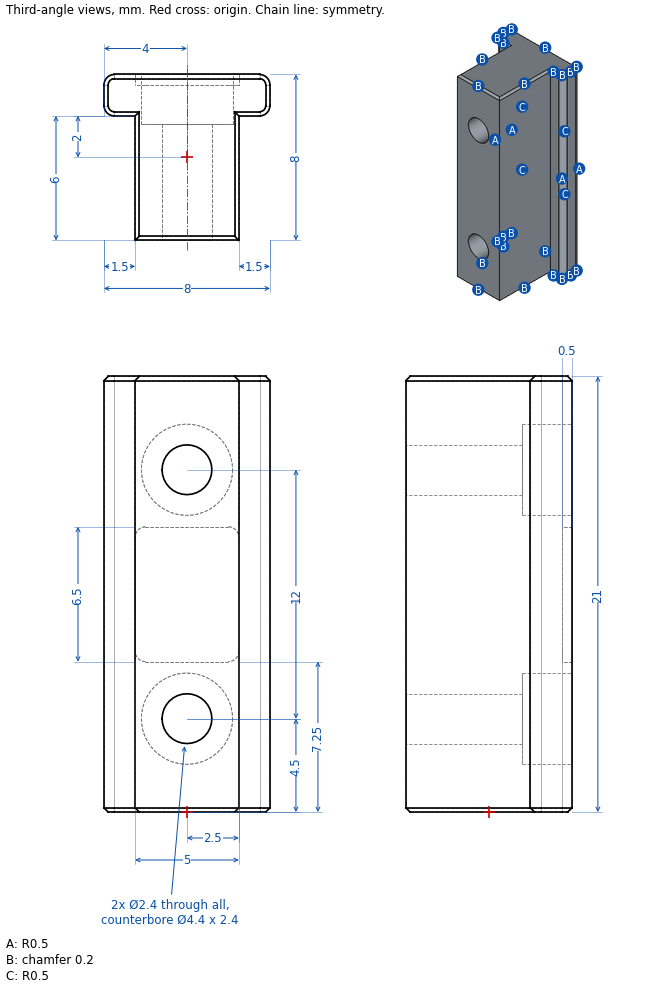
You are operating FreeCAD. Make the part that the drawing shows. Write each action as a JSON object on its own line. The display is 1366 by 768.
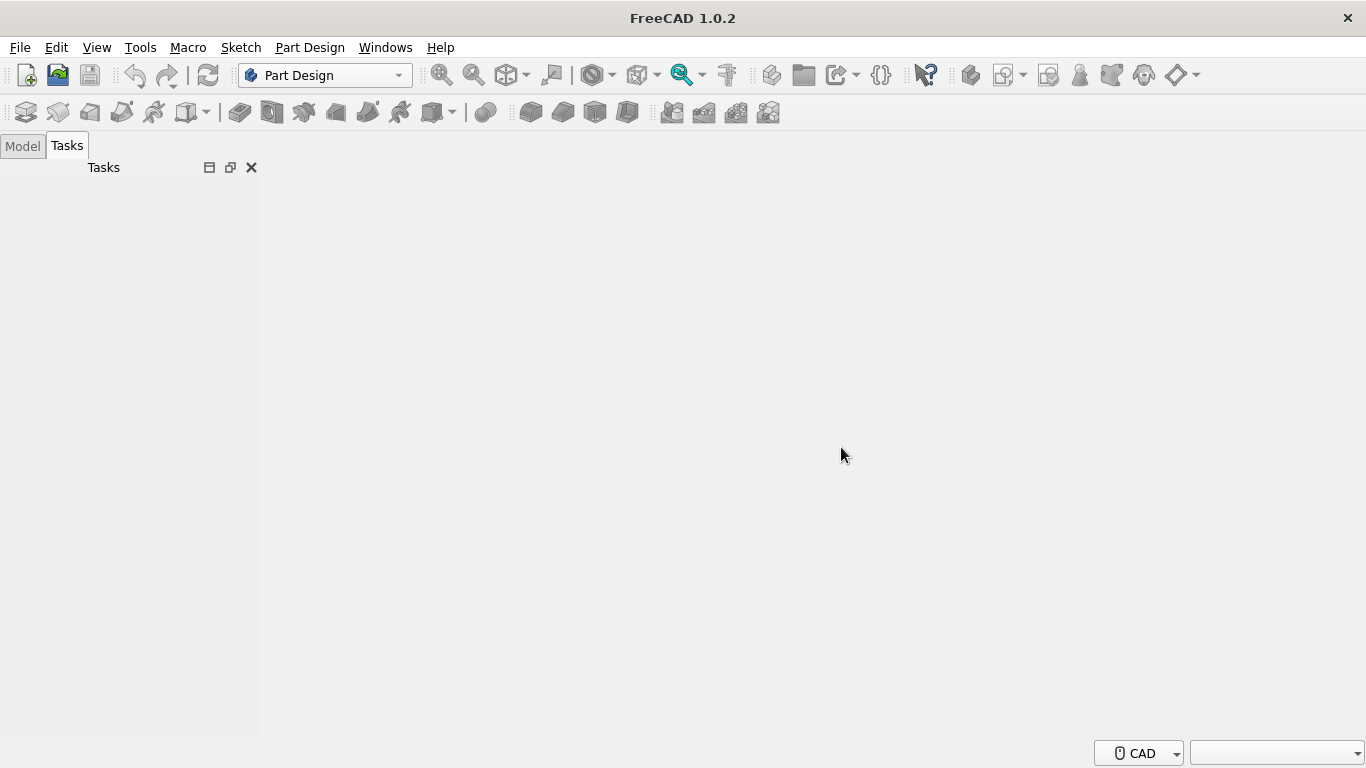
{"action": "left_click", "coordinate": [26, 76]}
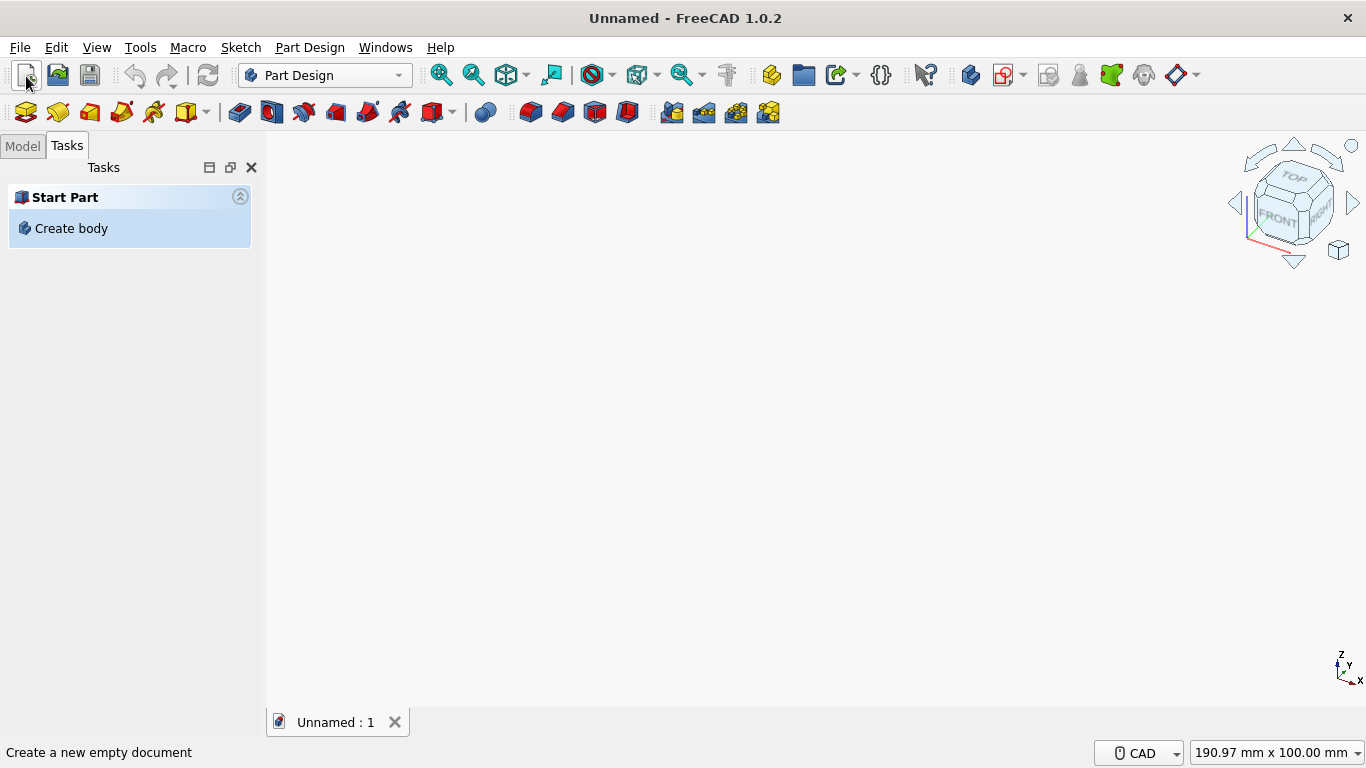
{"action": "left_click", "coordinate": [1004, 76]}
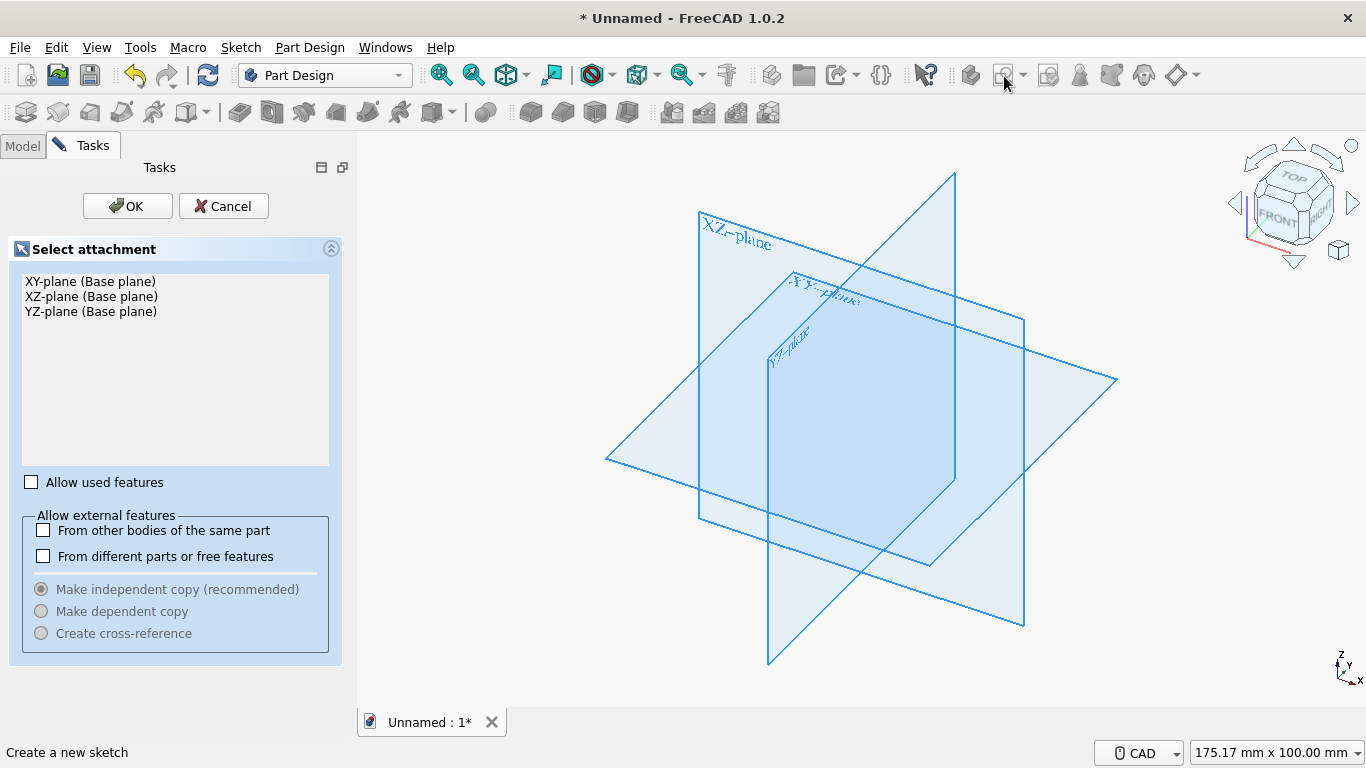
{"action": "left_click", "coordinate": [82, 282]}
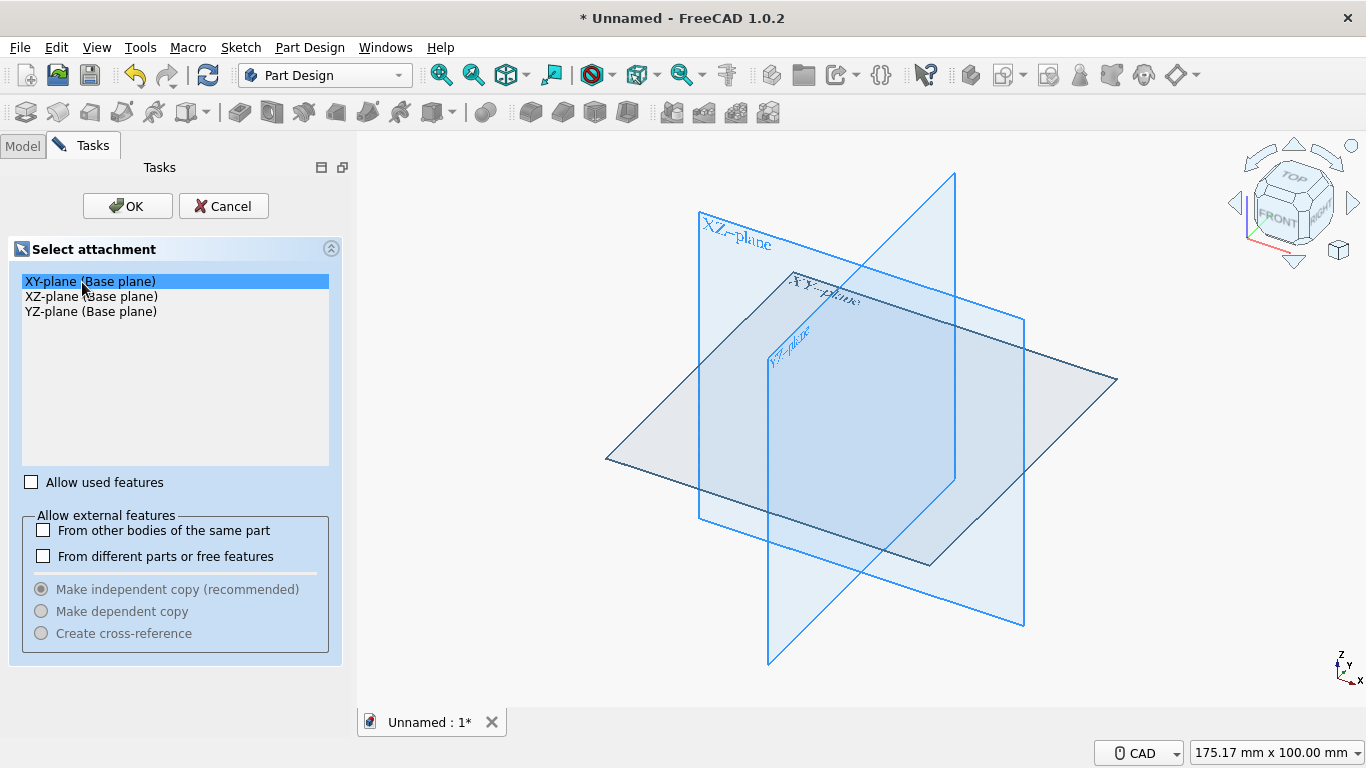
{"action": "left_click", "coordinate": [128, 206]}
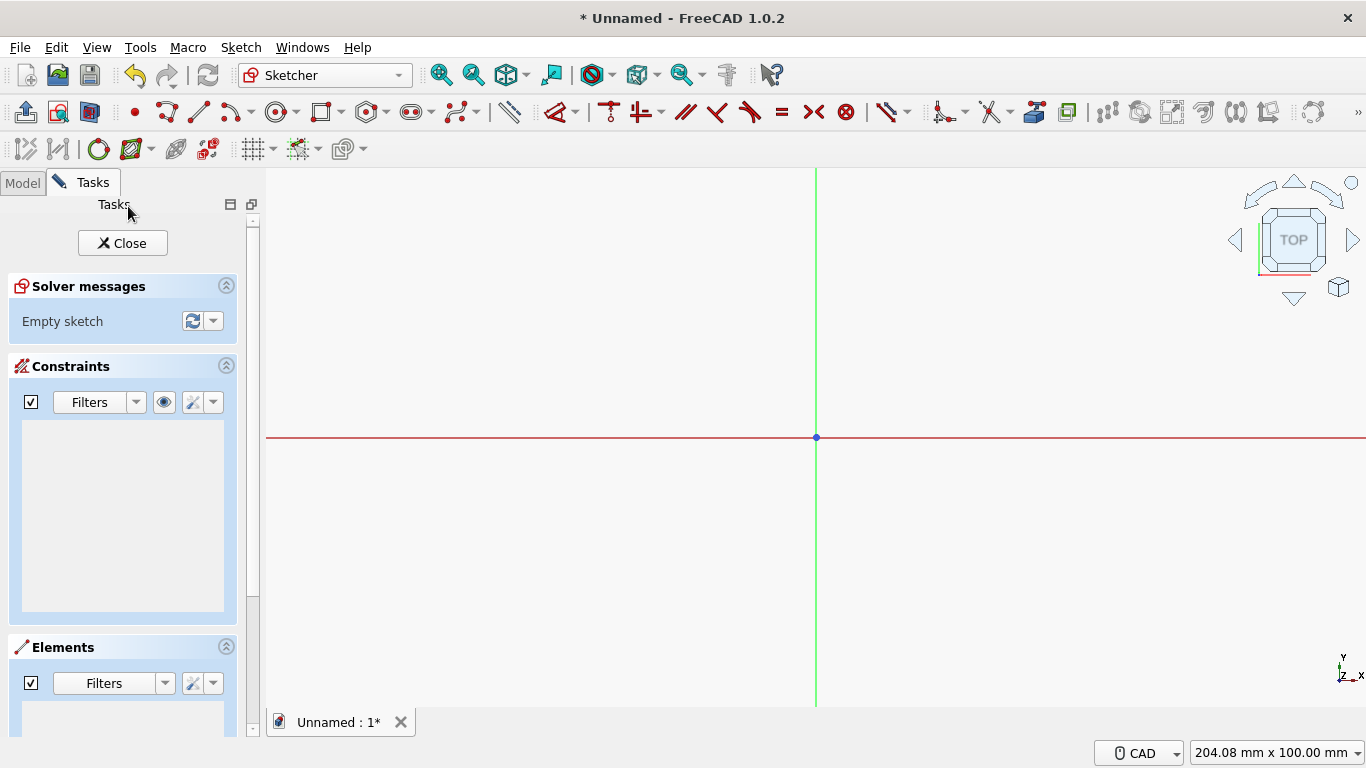
{"action": "scroll", "coordinate": [827, 437], "scroll_direction": "up", "scroll_amount": 10}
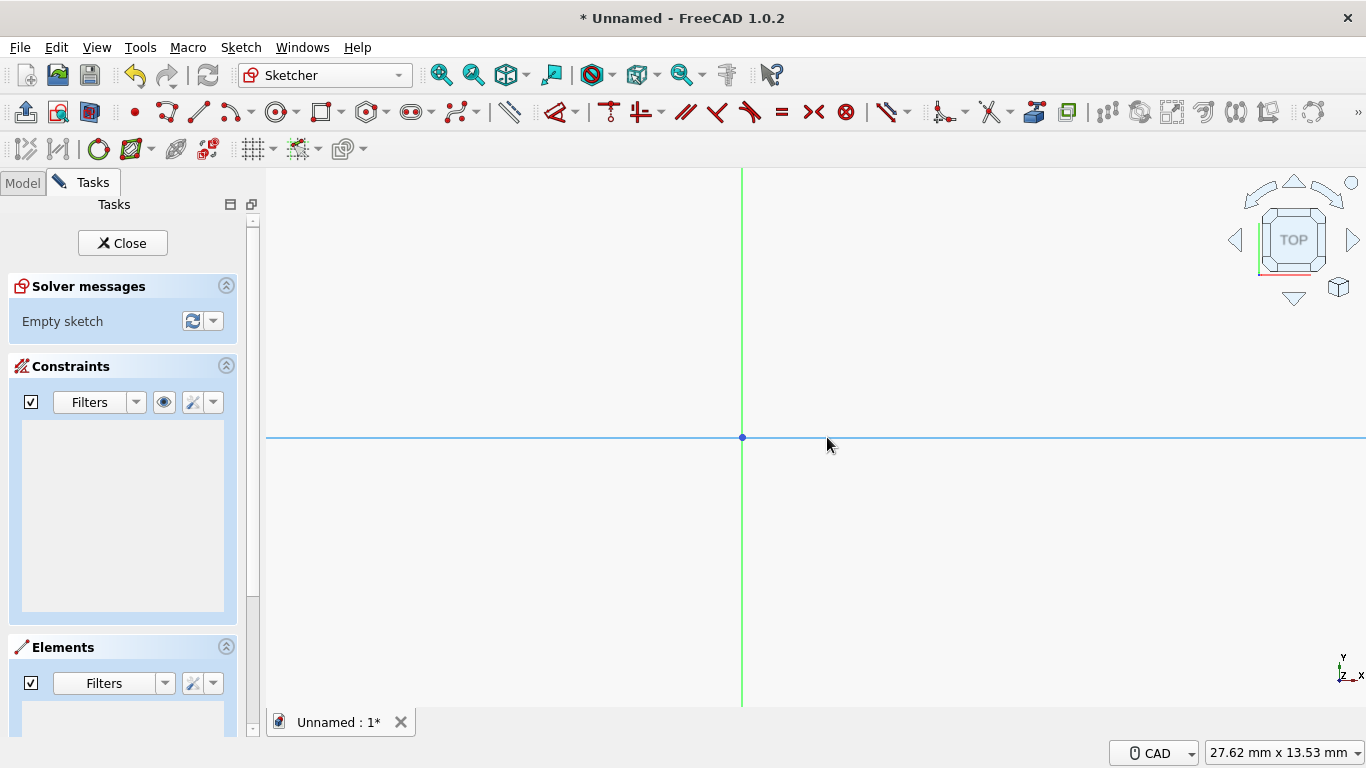
{"action": "key", "text": "g v"}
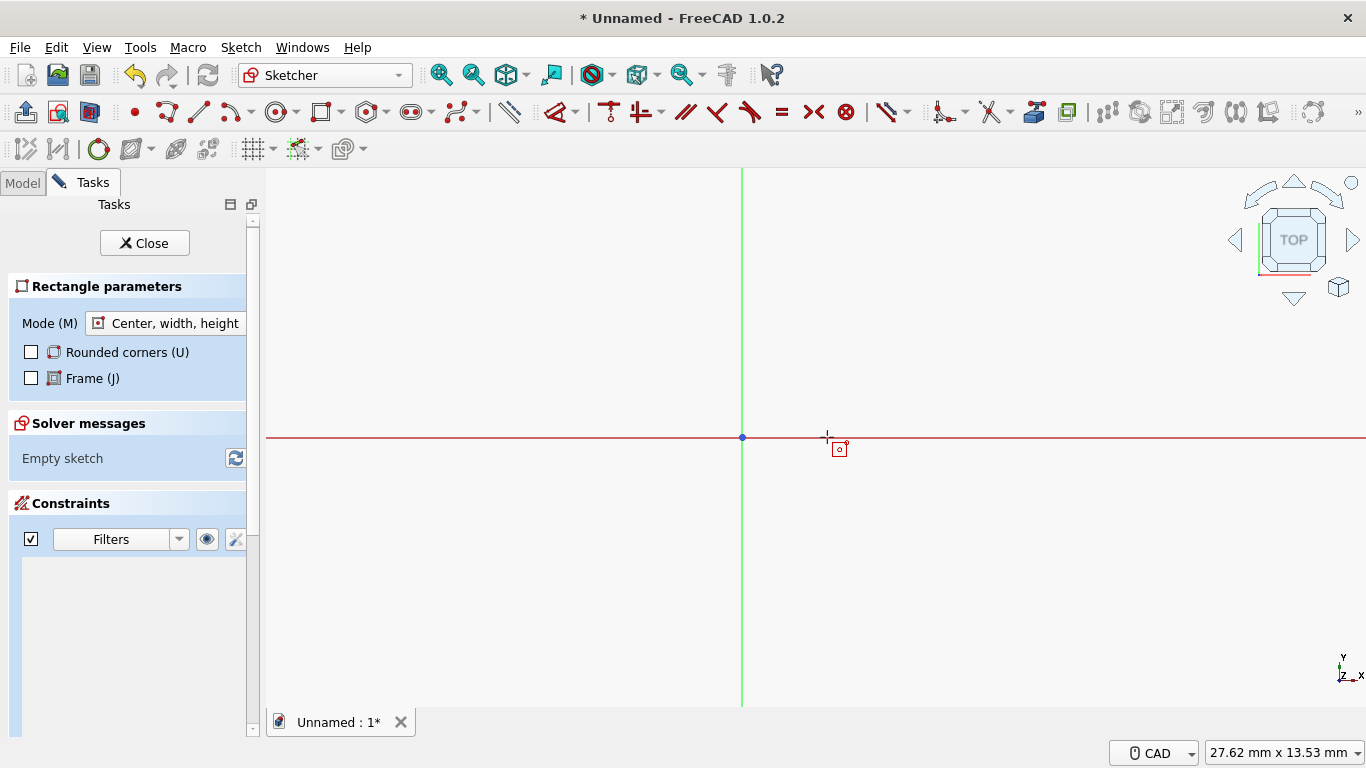
{"action": "left_click", "coordinate": [742, 438]}
{"action": "mouse_move", "coordinate": [902, 278]}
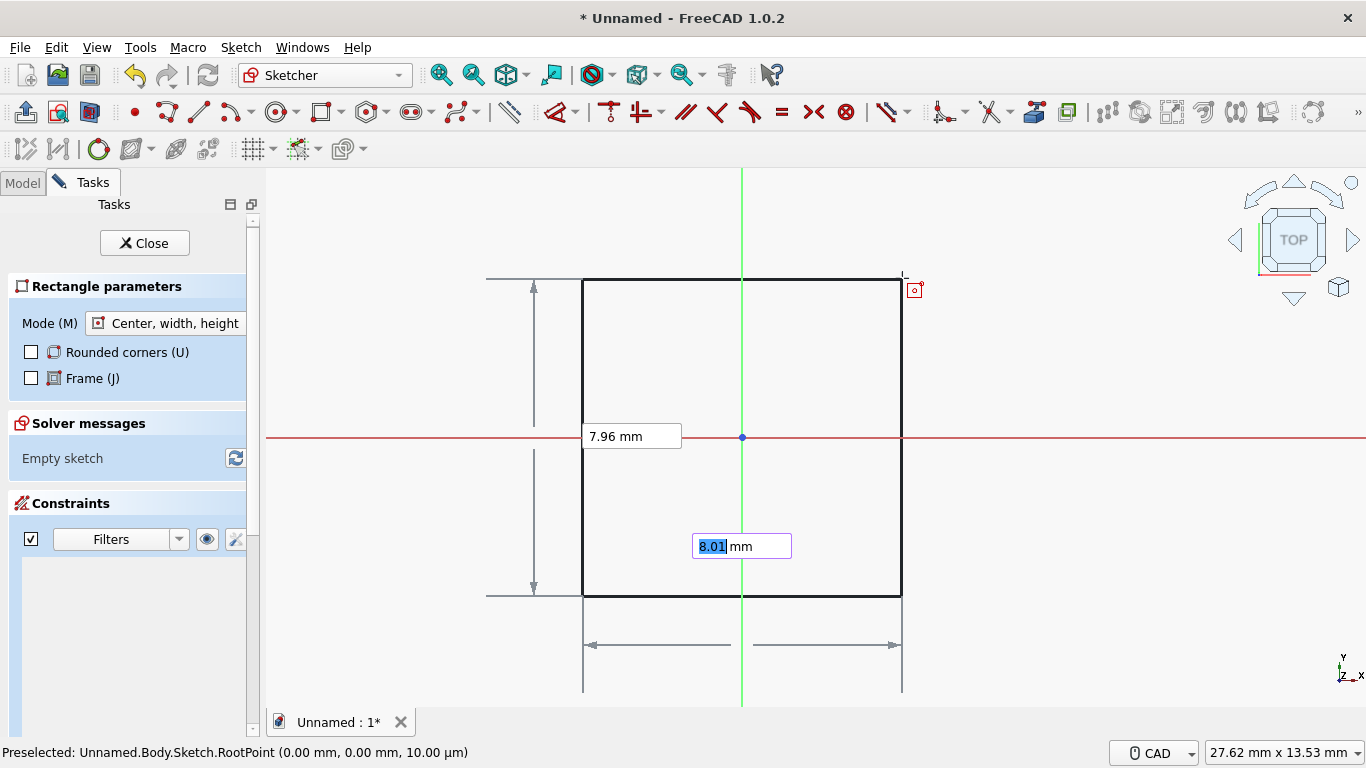
{"action": "type", "text": "8"}
{"action": "key", "text": "Tab"}
{"action": "type", "text": "8"}
{"action": "key", "text": "Return"}
{"action": "key", "text": "Escape"}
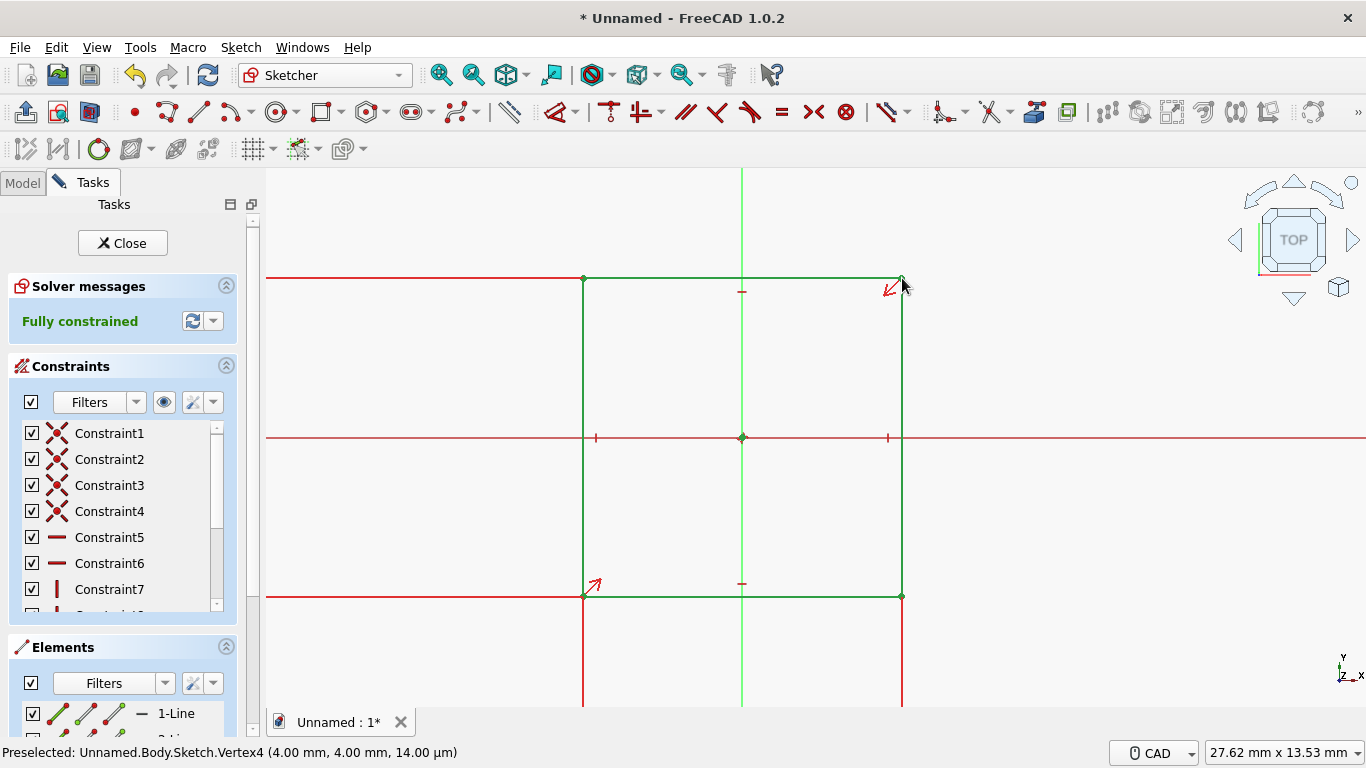
{"action": "left_click", "coordinate": [123, 243]}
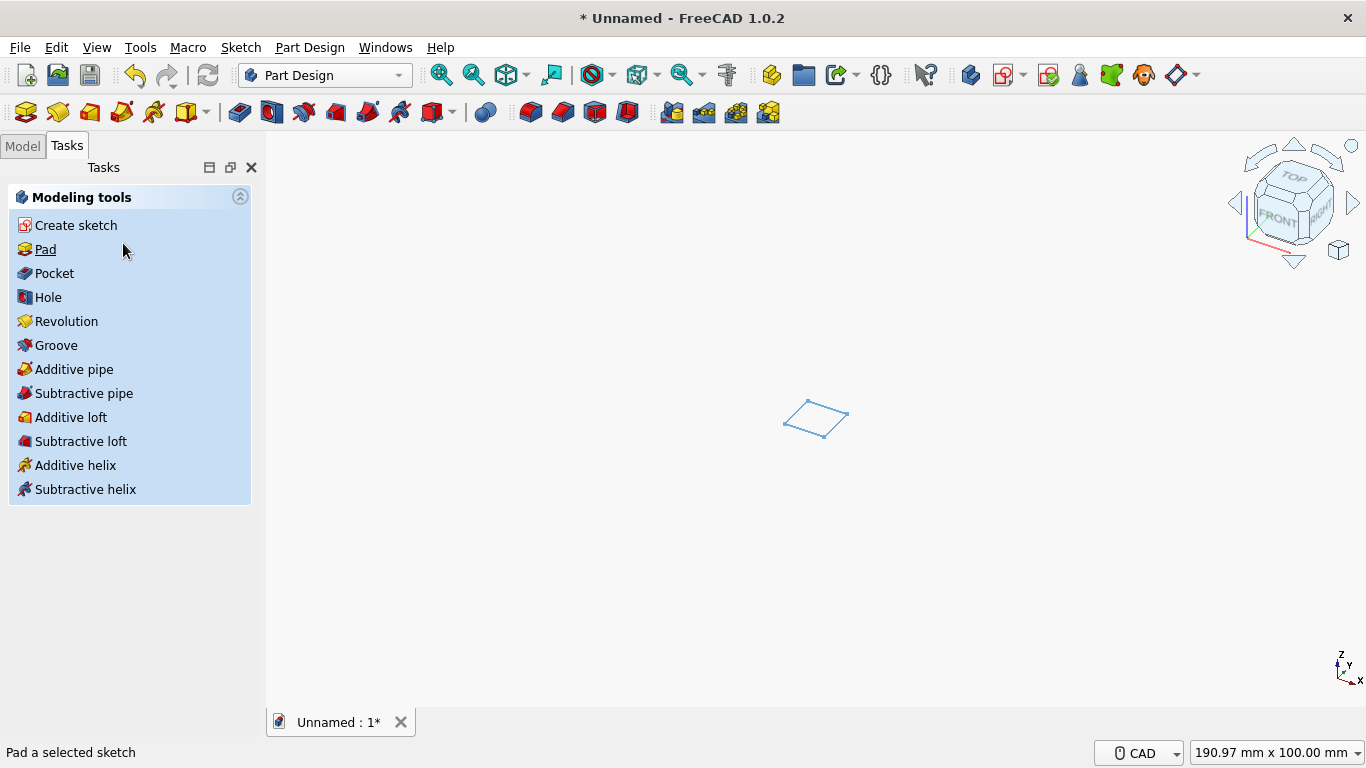
{"action": "left_click", "coordinate": [26, 112]}